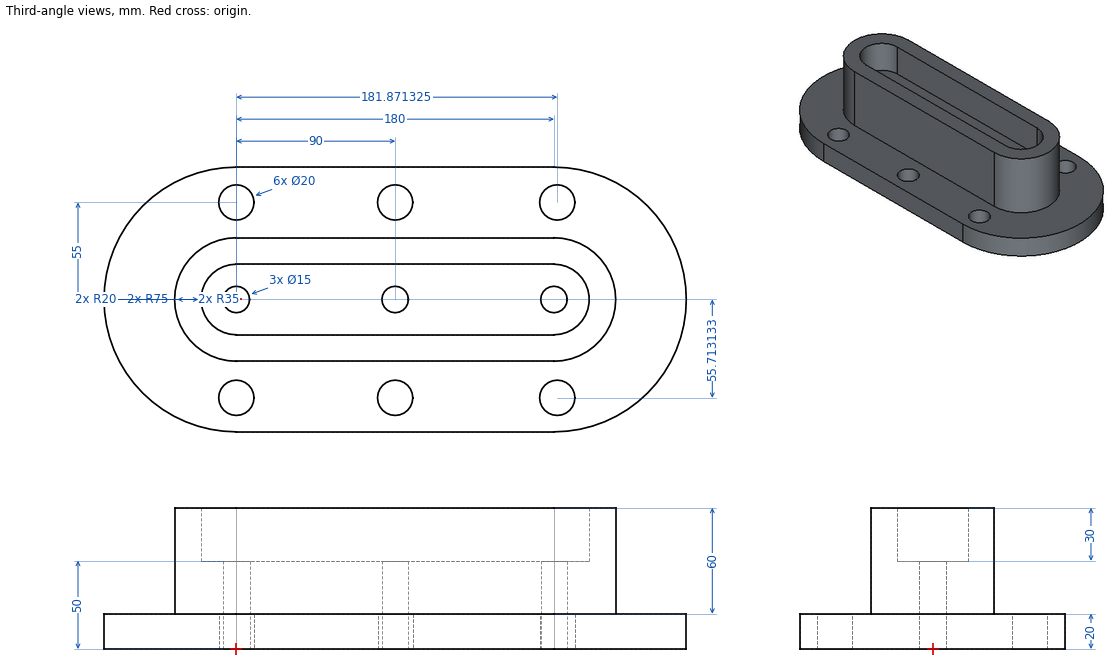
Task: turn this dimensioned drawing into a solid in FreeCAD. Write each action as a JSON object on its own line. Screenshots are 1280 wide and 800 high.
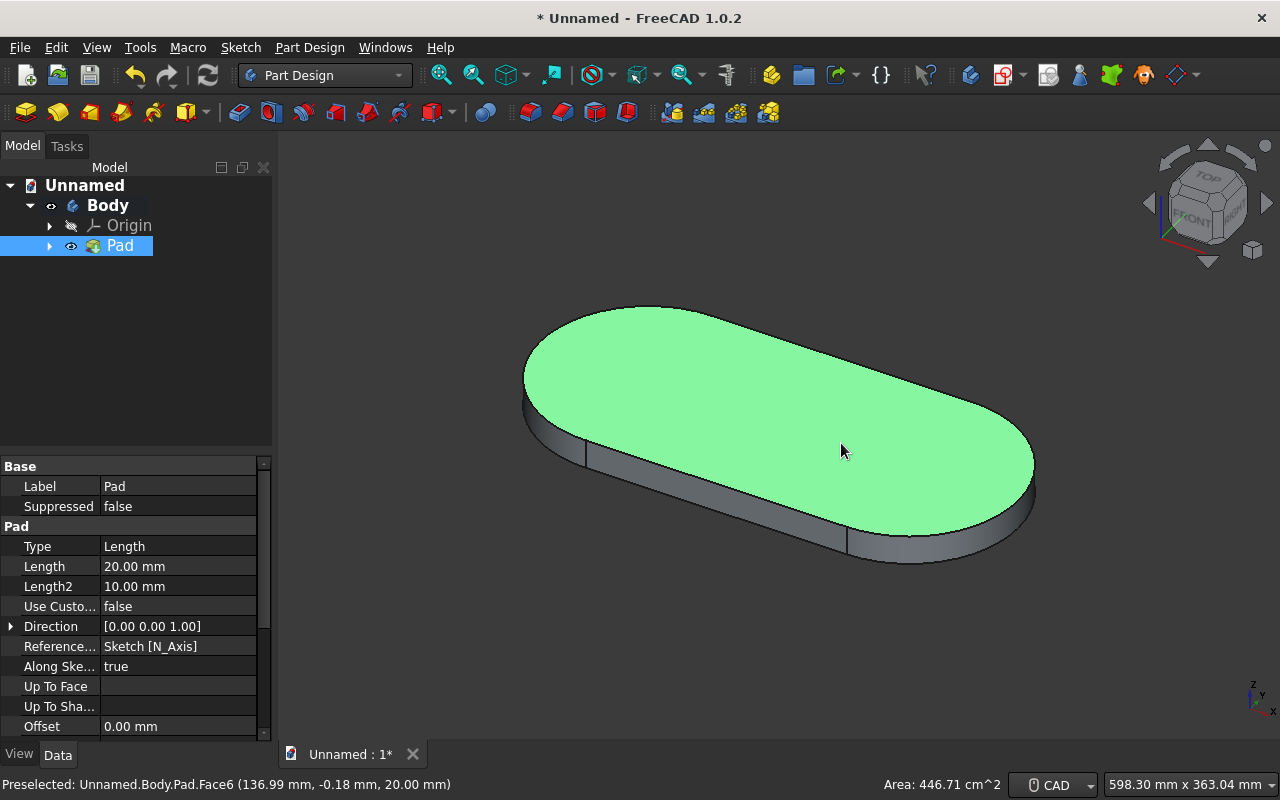
{"action": "left_click", "coordinate": [1004, 76]}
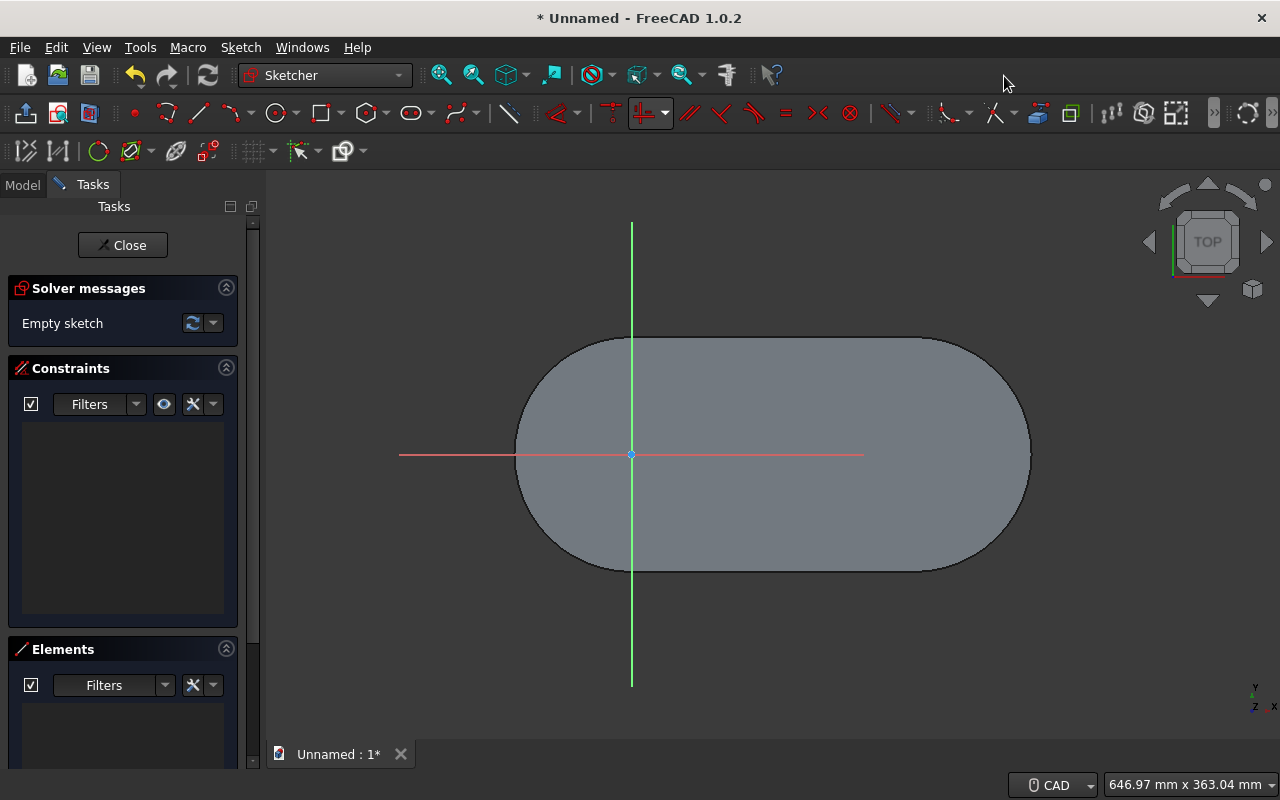
{"action": "scroll", "coordinate": [912, 455], "scroll_direction": "up", "scroll_amount": 2}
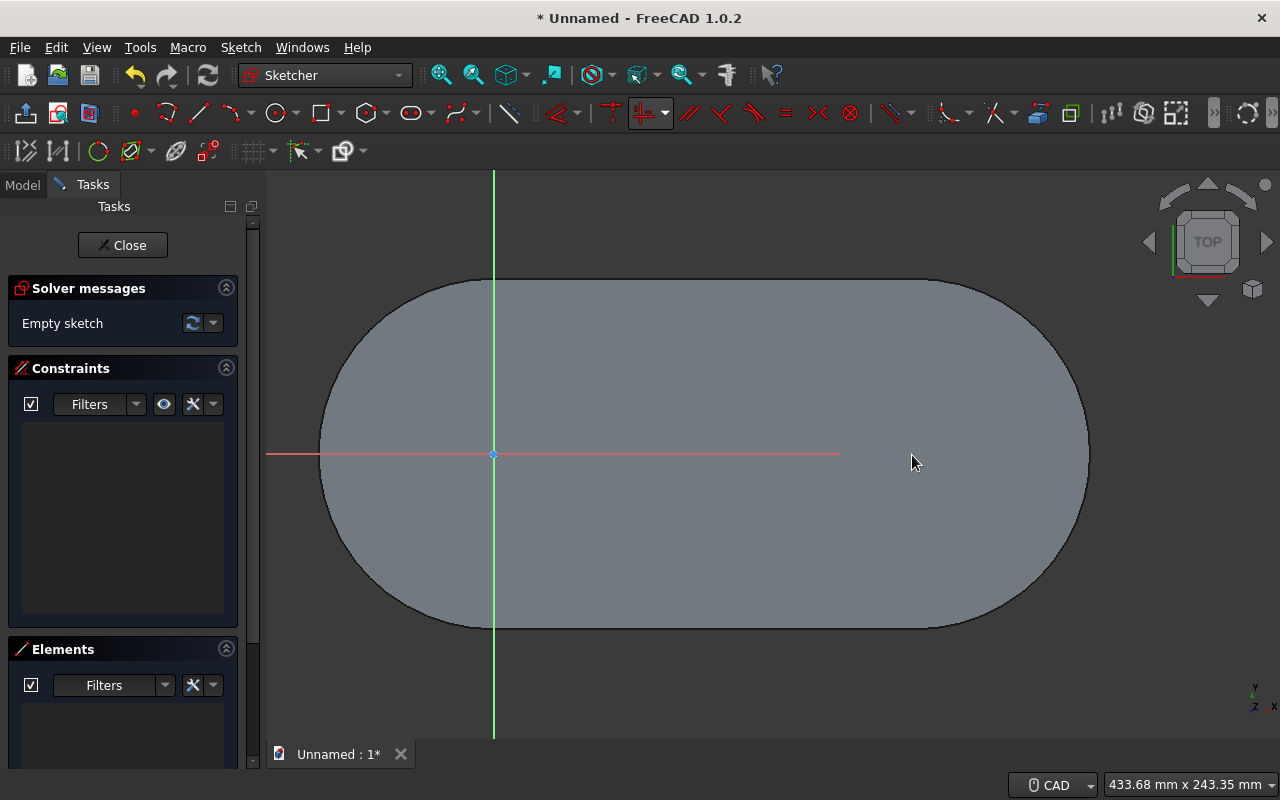
{"action": "key", "text": "g s"}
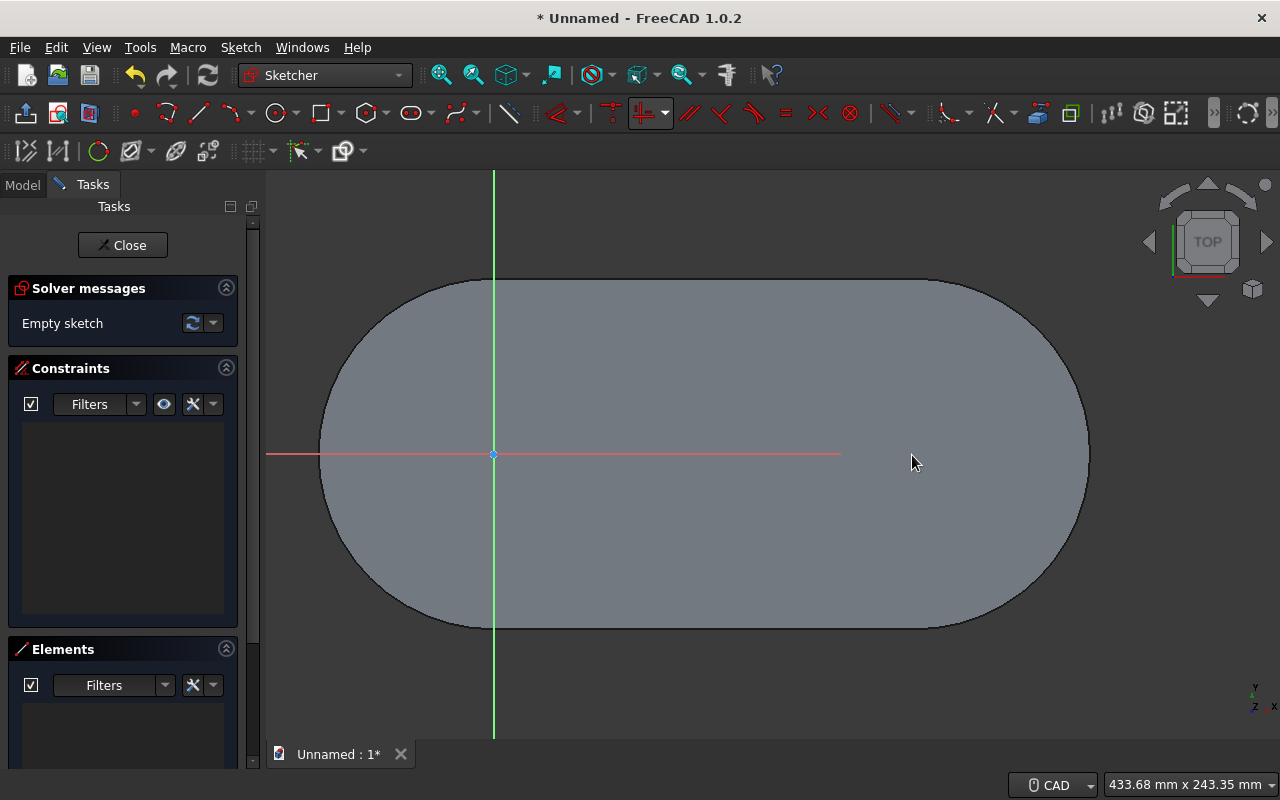
{"action": "left_click", "coordinate": [494, 454]}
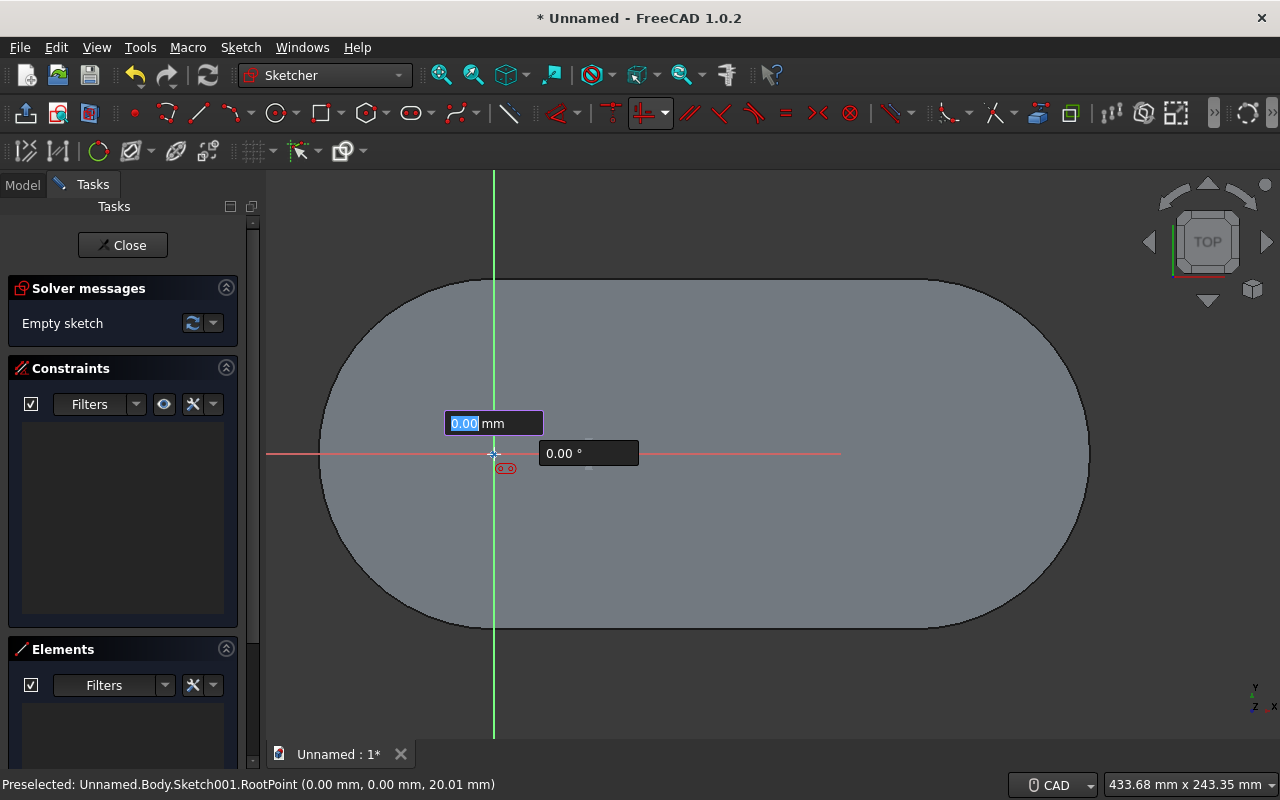
{"action": "left_click", "coordinate": [915, 445]}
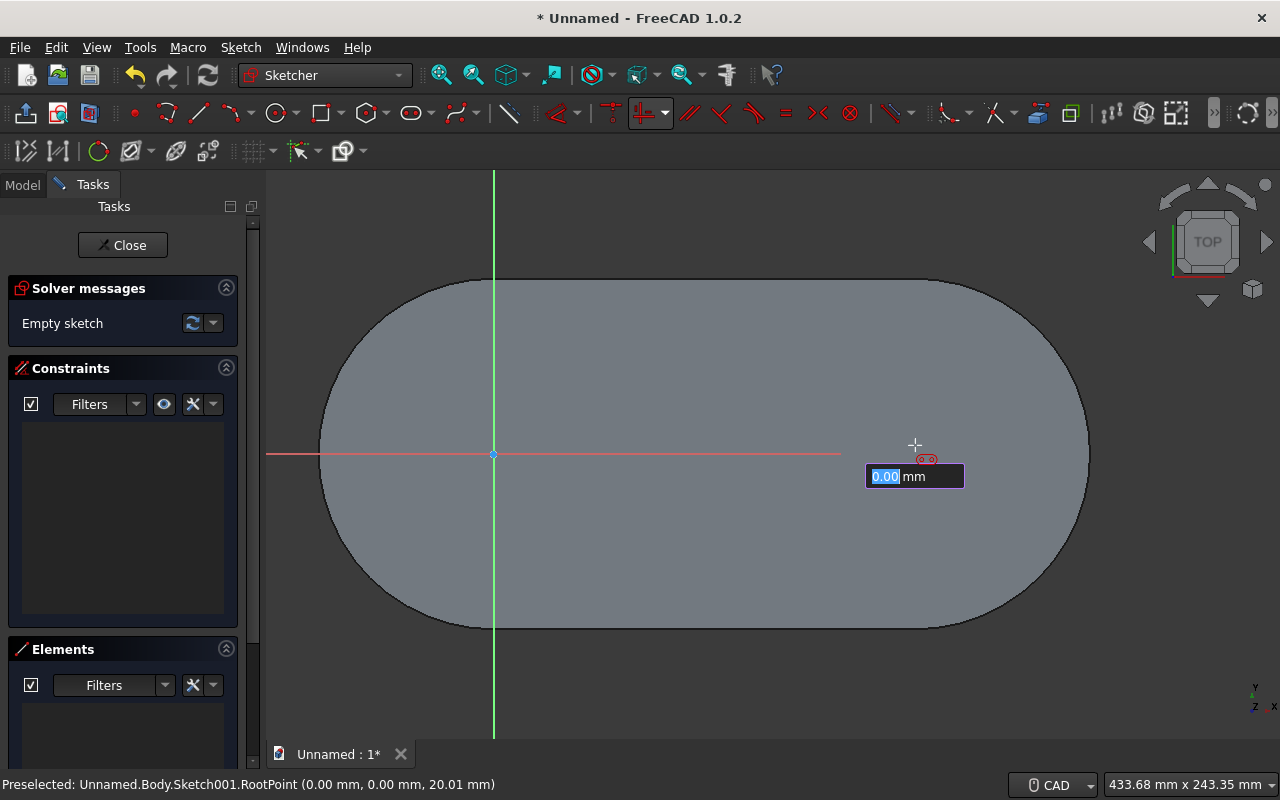
{"action": "left_click", "coordinate": [704, 372]}
{"action": "key", "text": "Escape"}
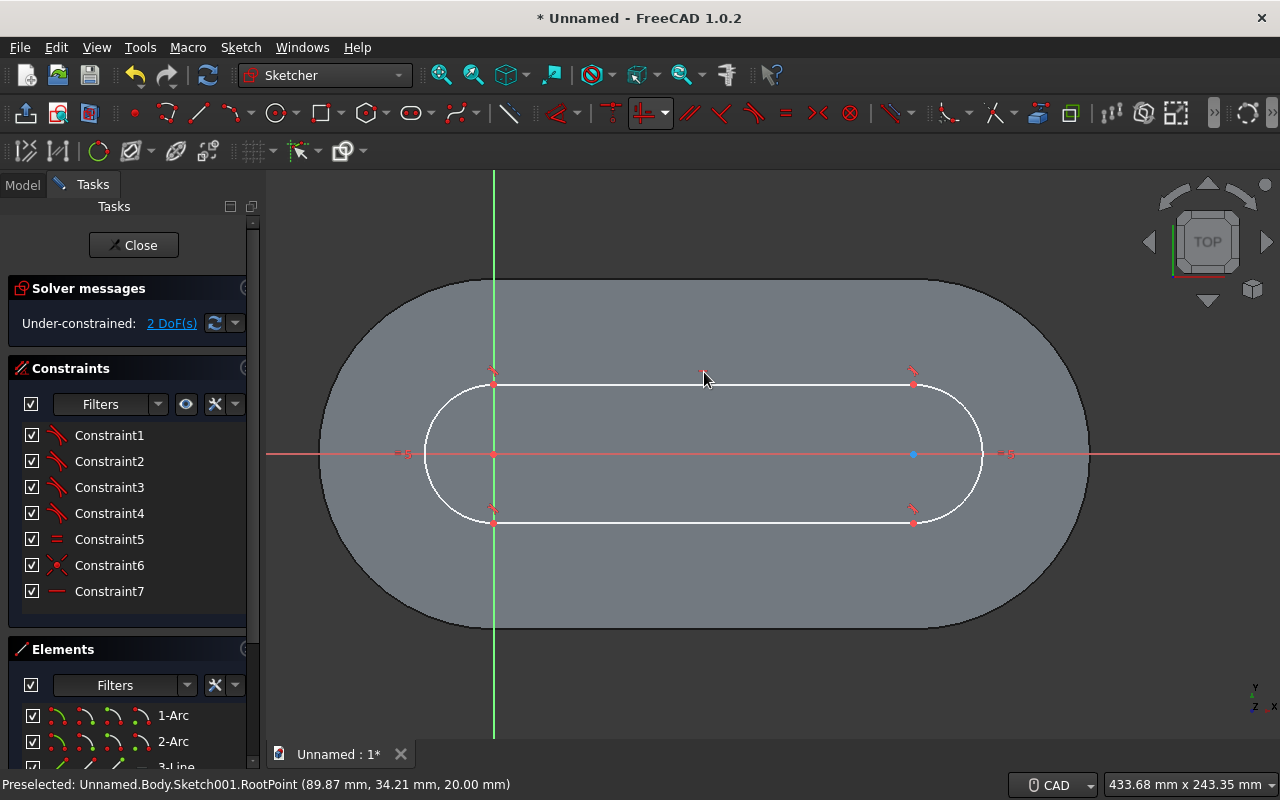
{"action": "left_click", "coordinate": [556, 114]}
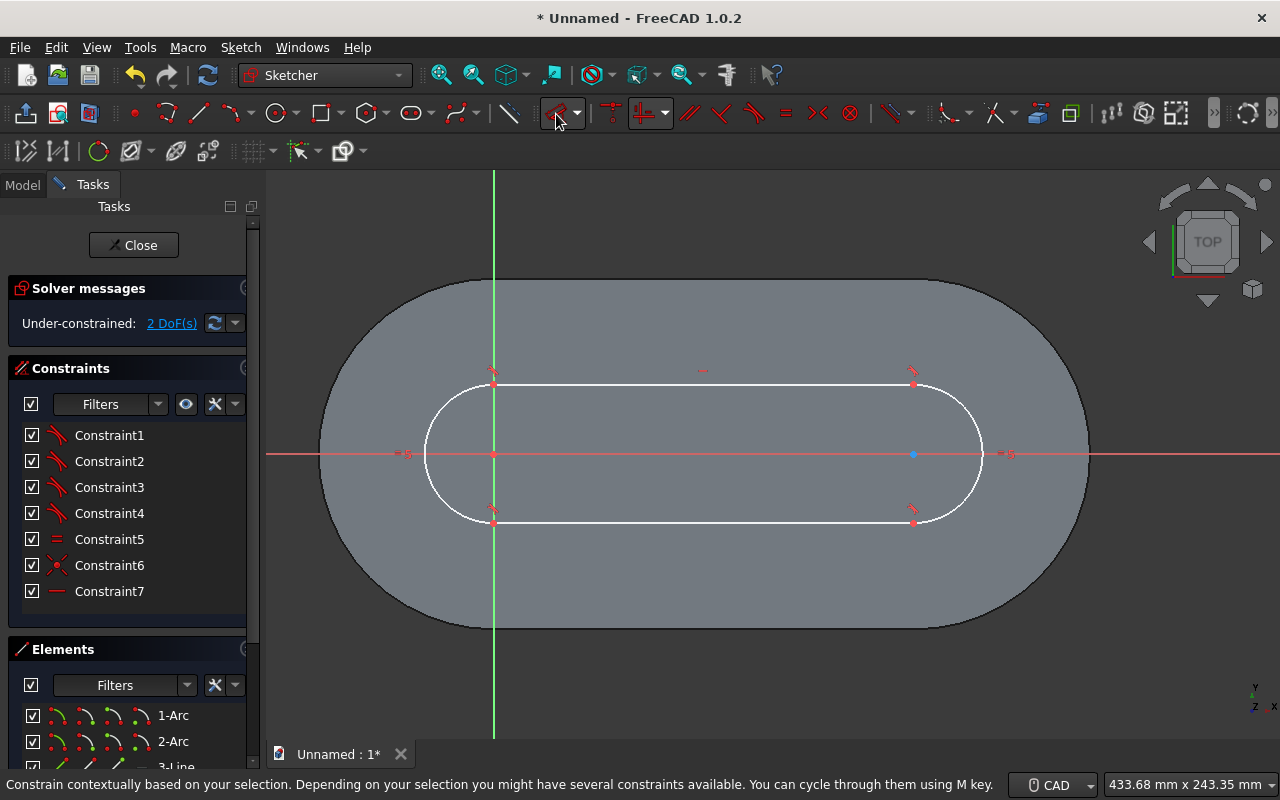
{"action": "left_click", "coordinate": [438, 413]}
{"action": "left_click", "coordinate": [412, 394]}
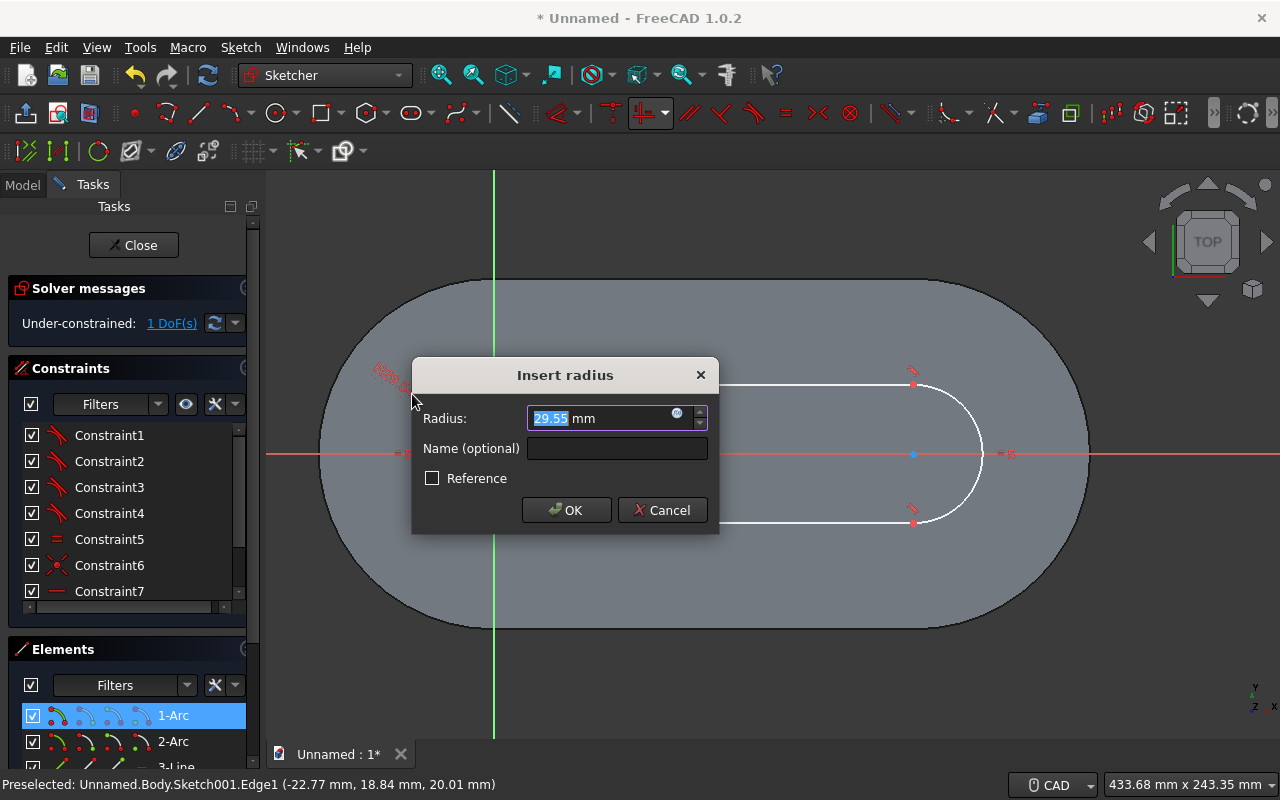
{"action": "type", "text": "35"}
{"action": "key", "text": "Return"}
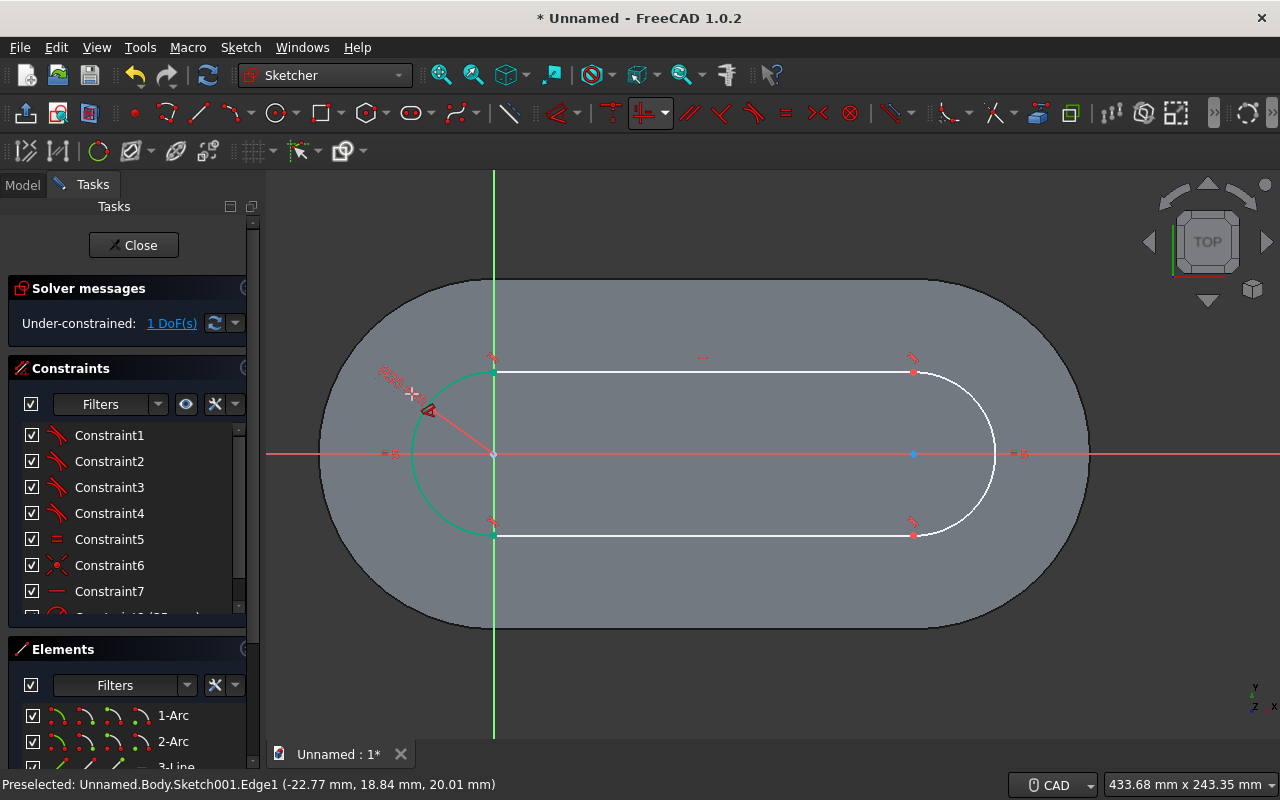
{"action": "left_click", "coordinate": [620, 372]}
{"action": "left_click", "coordinate": [704, 338]}